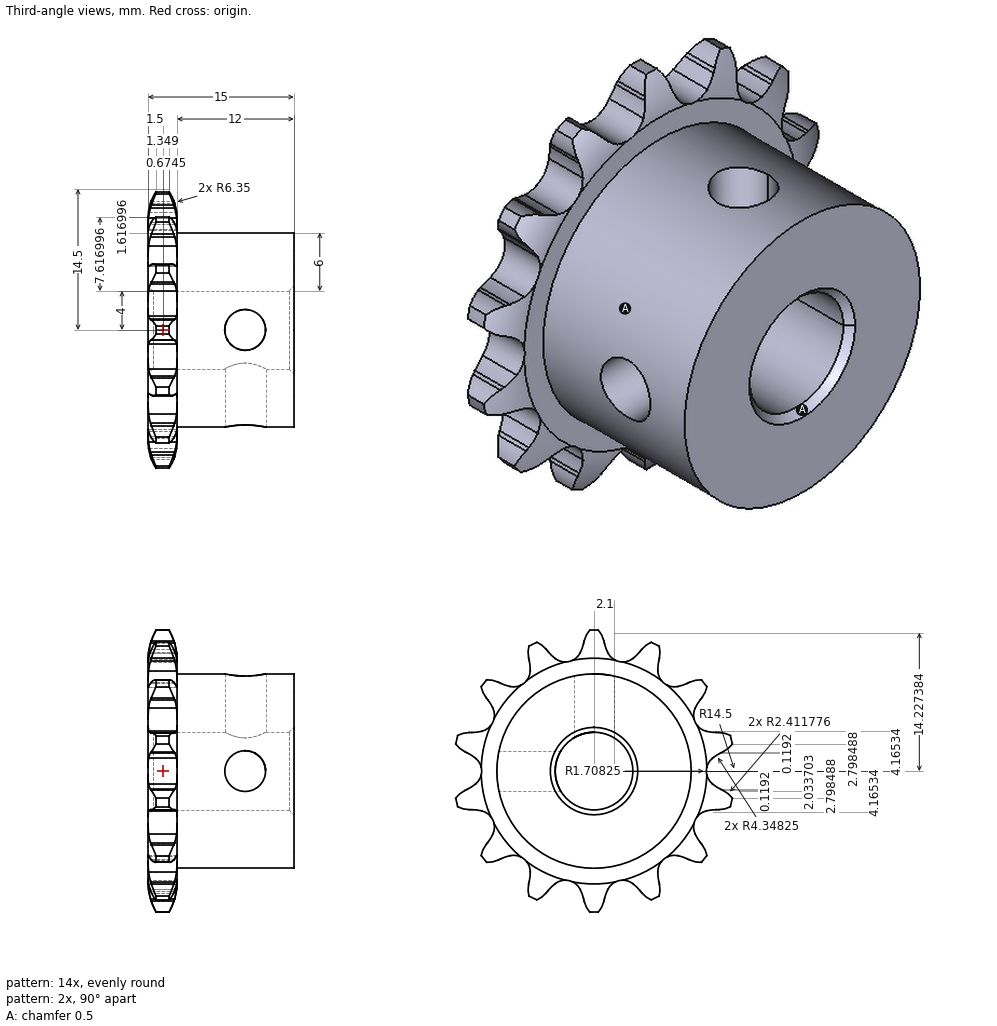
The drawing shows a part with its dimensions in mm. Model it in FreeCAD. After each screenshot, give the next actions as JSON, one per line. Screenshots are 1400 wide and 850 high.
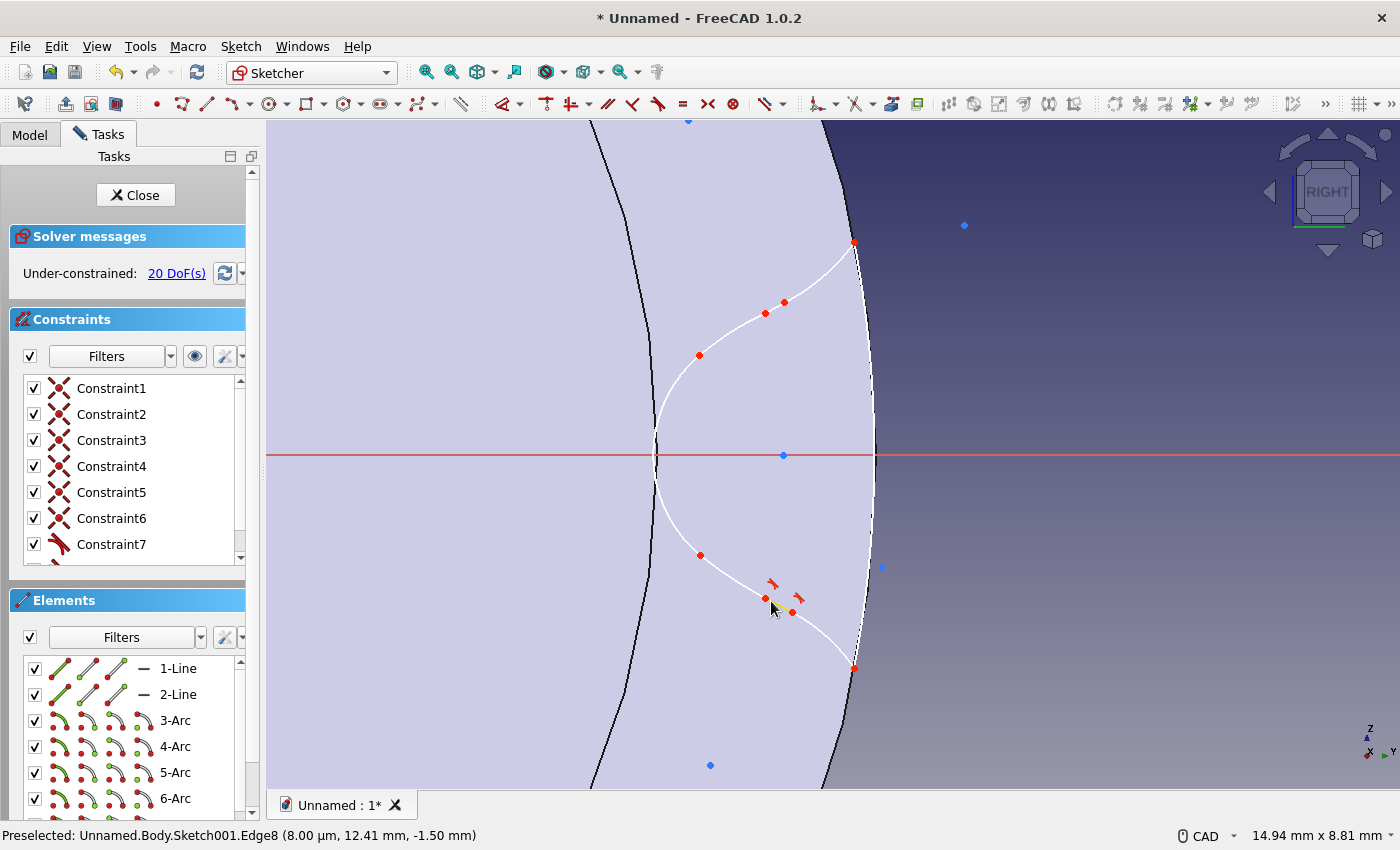
{"action": "scroll", "coordinate": [779, 306], "scroll_direction": "up", "scroll_amount": 4}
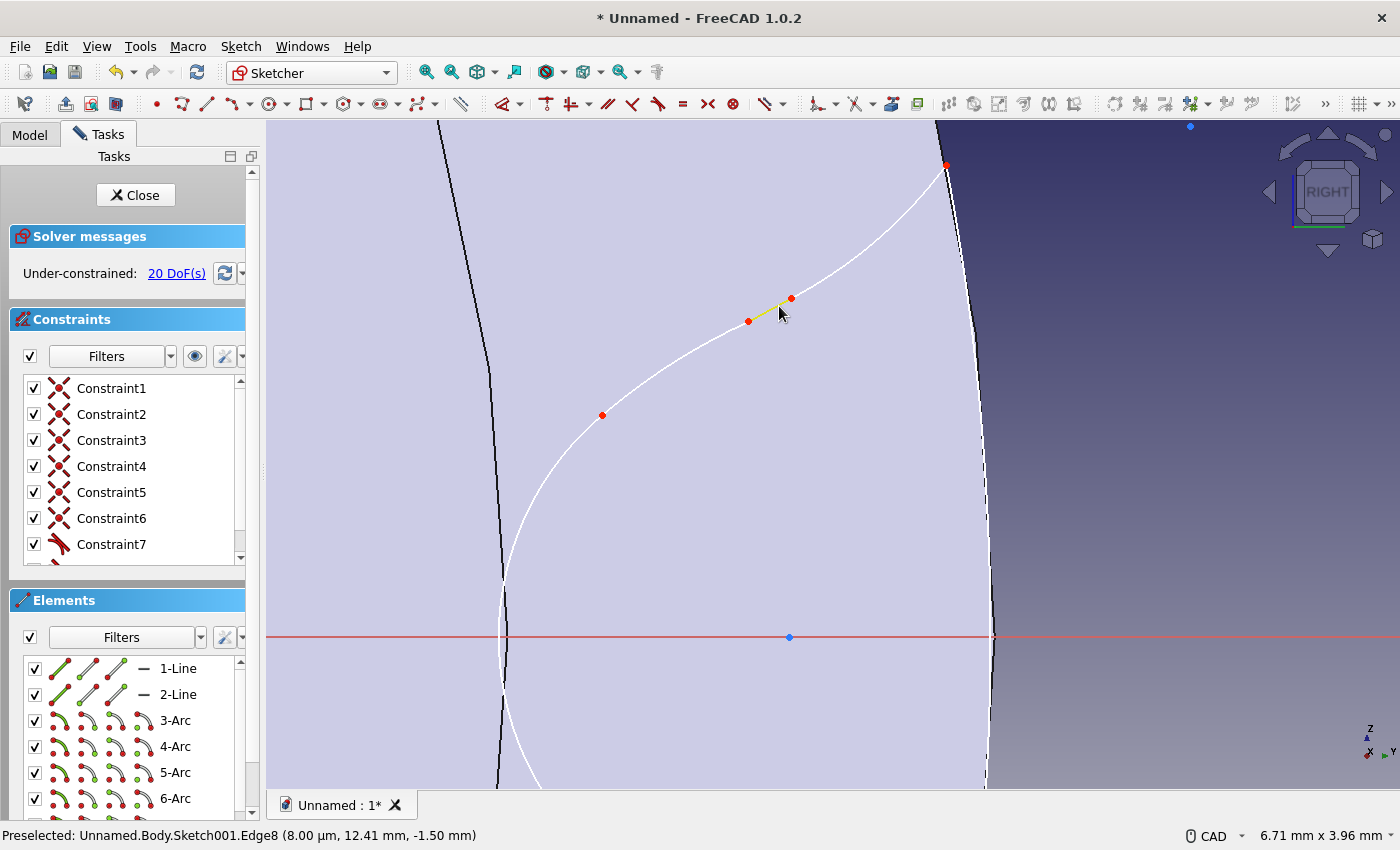
{"action": "left_click", "coordinate": [778, 306]}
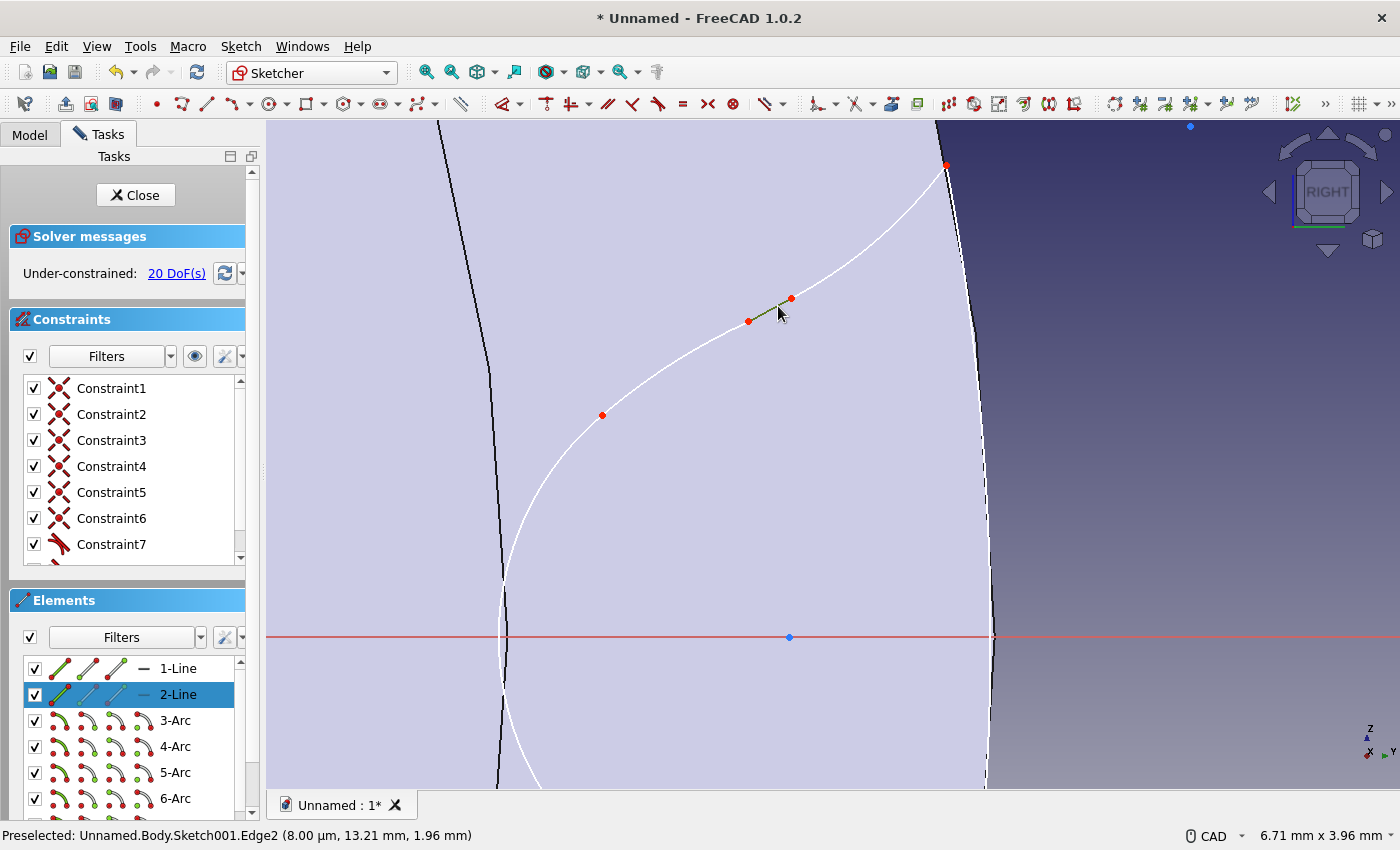
{"action": "left_click", "coordinate": [844, 266]}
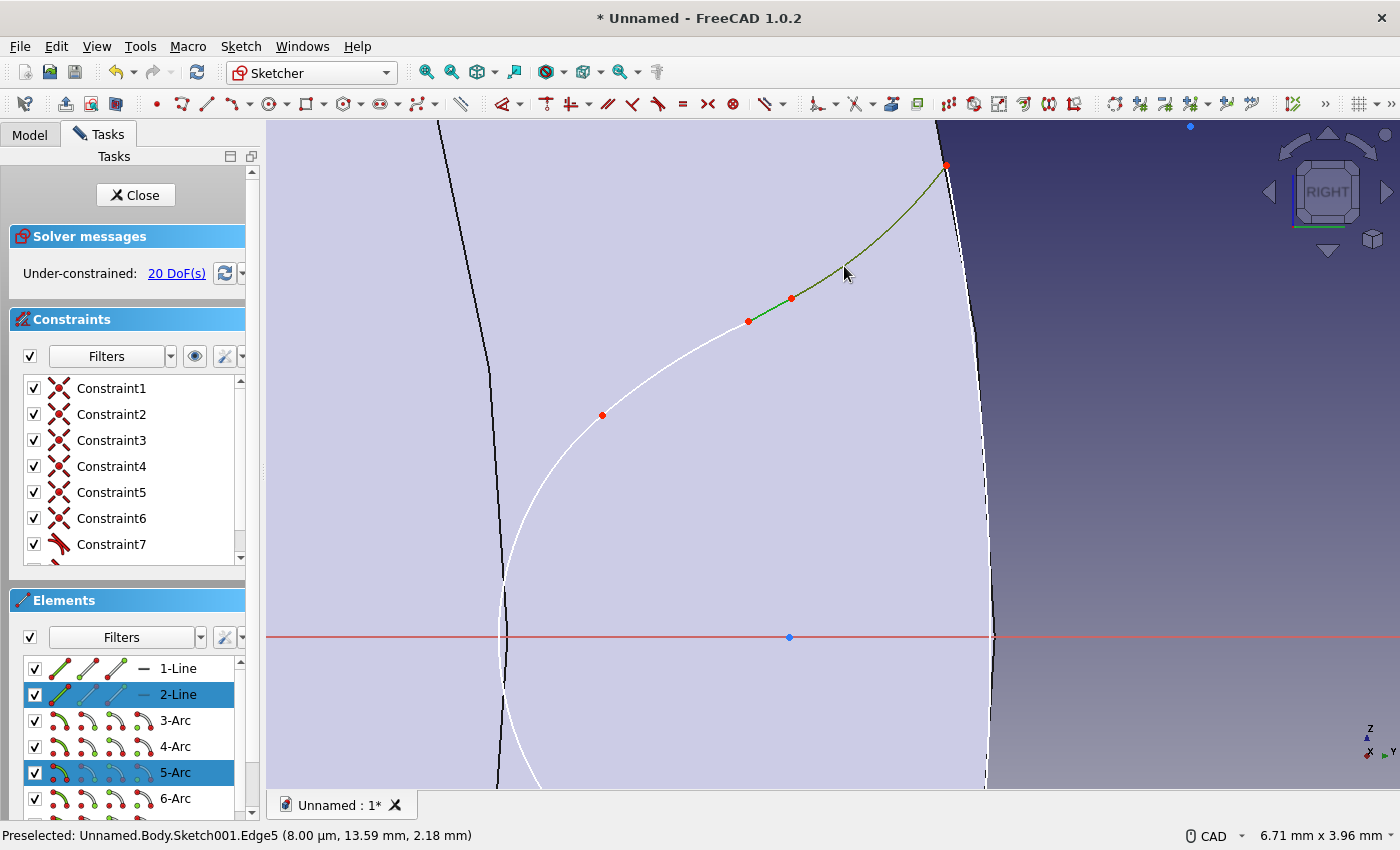
{"action": "left_click", "coordinate": [658, 104]}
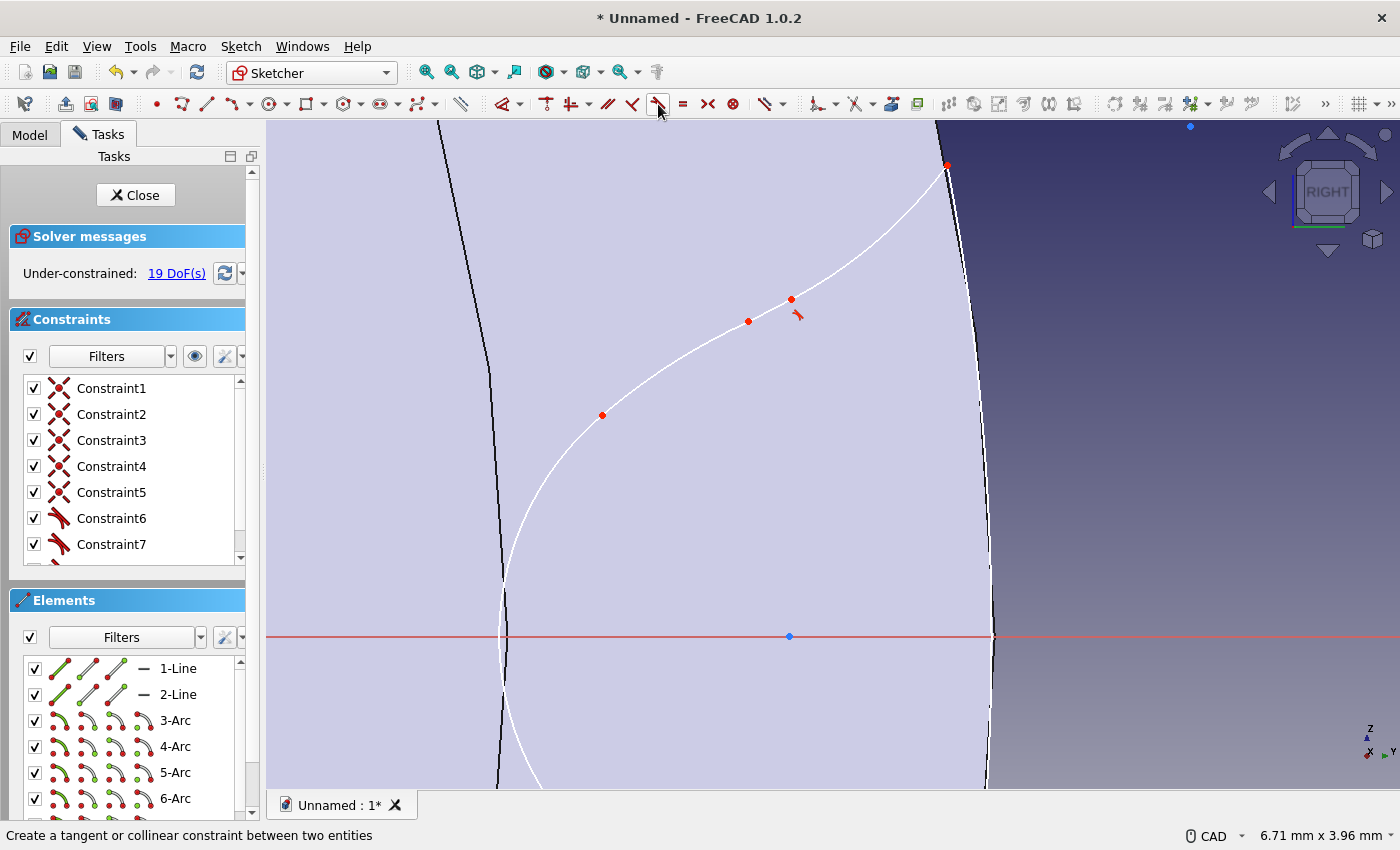
{"action": "left_click", "coordinate": [778, 306]}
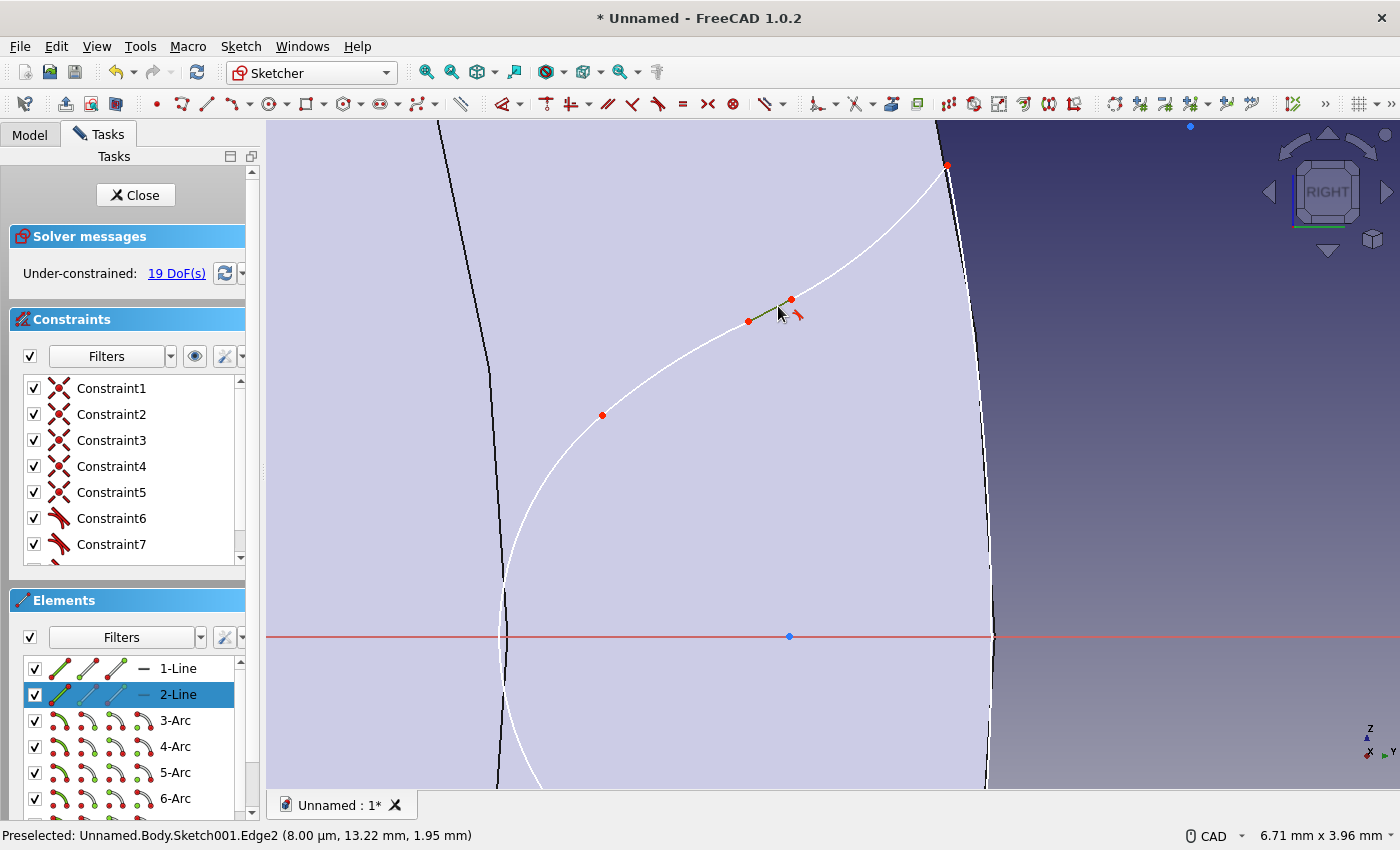
{"action": "left_click", "coordinate": [702, 345]}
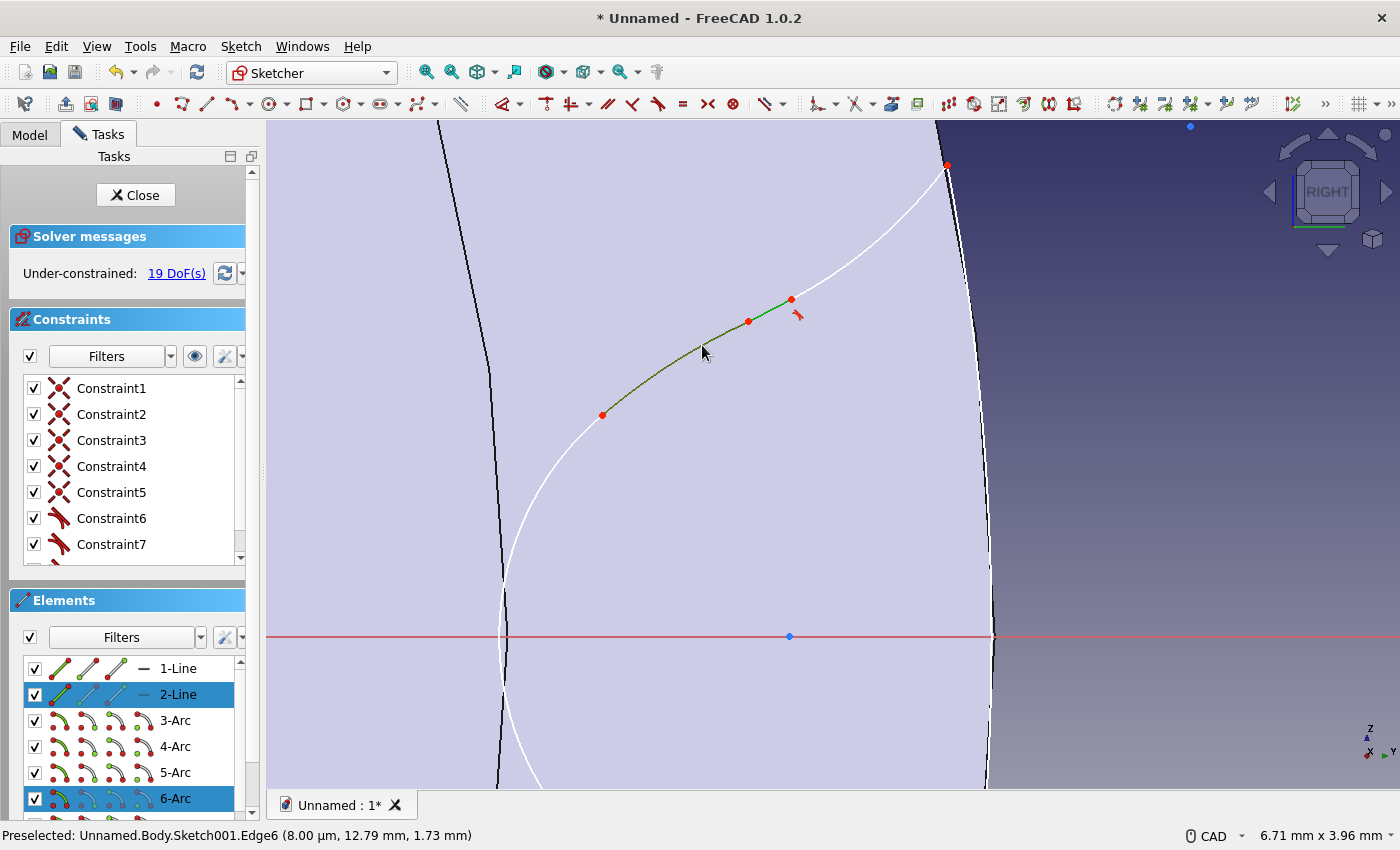
{"action": "left_click", "coordinate": [658, 104]}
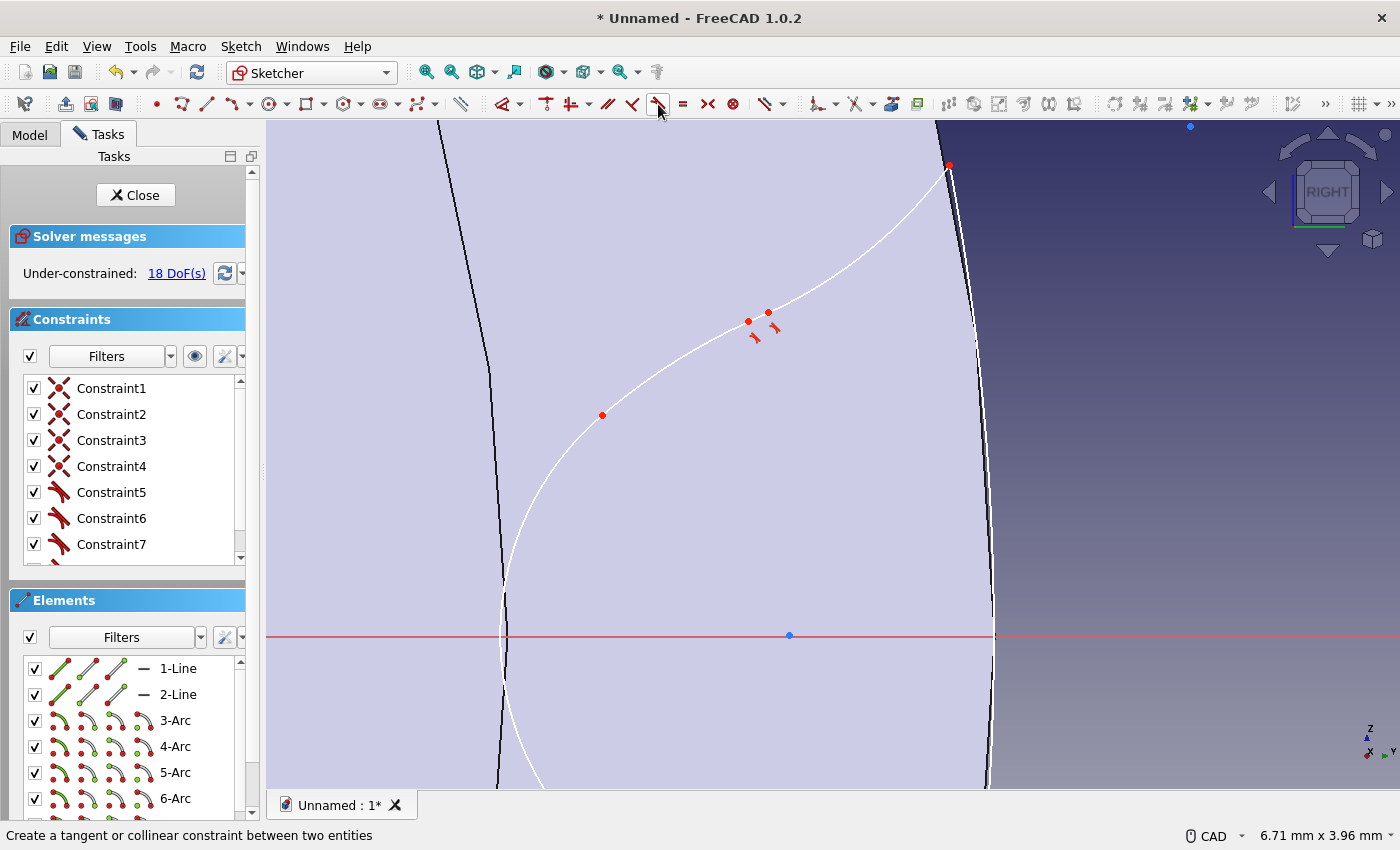
{"action": "left_click", "coordinate": [702, 346]}